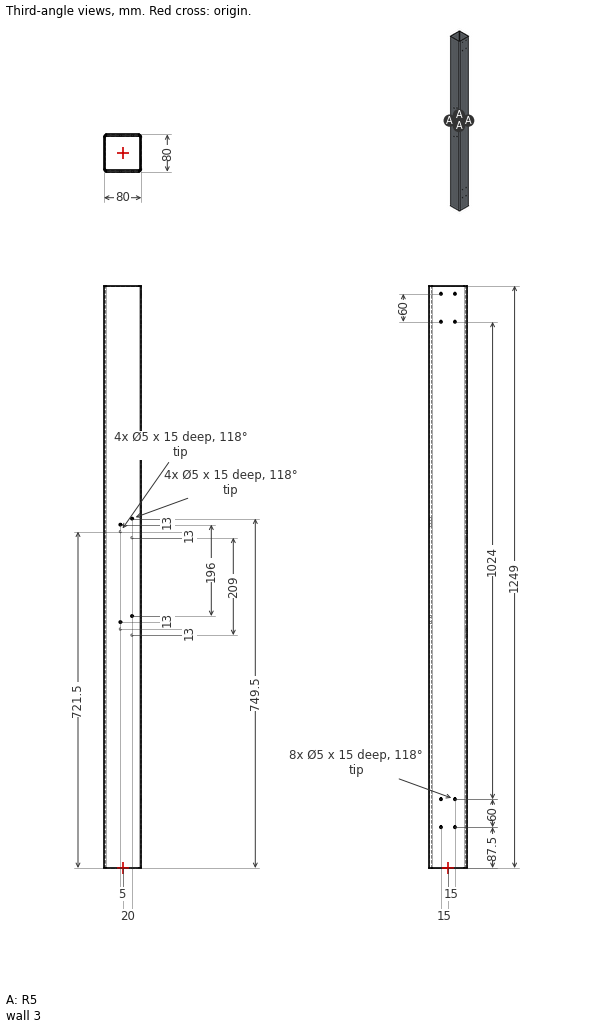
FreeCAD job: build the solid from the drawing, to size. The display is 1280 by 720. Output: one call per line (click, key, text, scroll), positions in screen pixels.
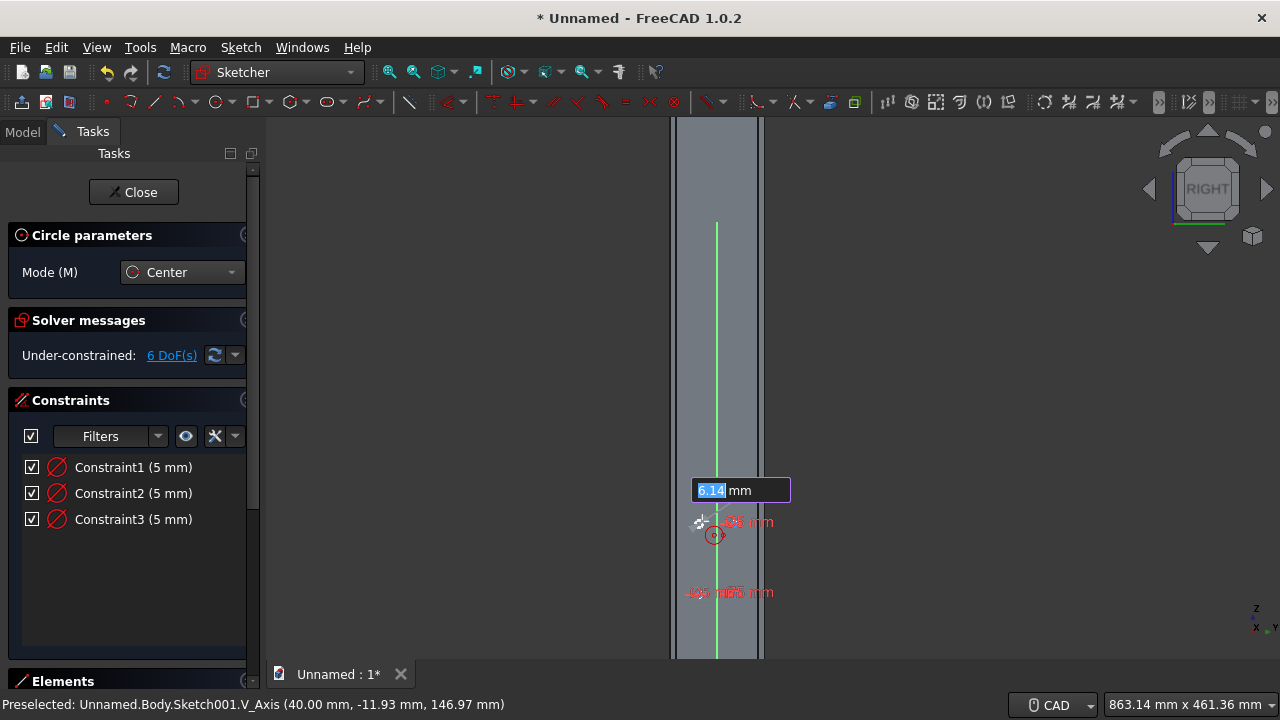
text(5)
key(Return)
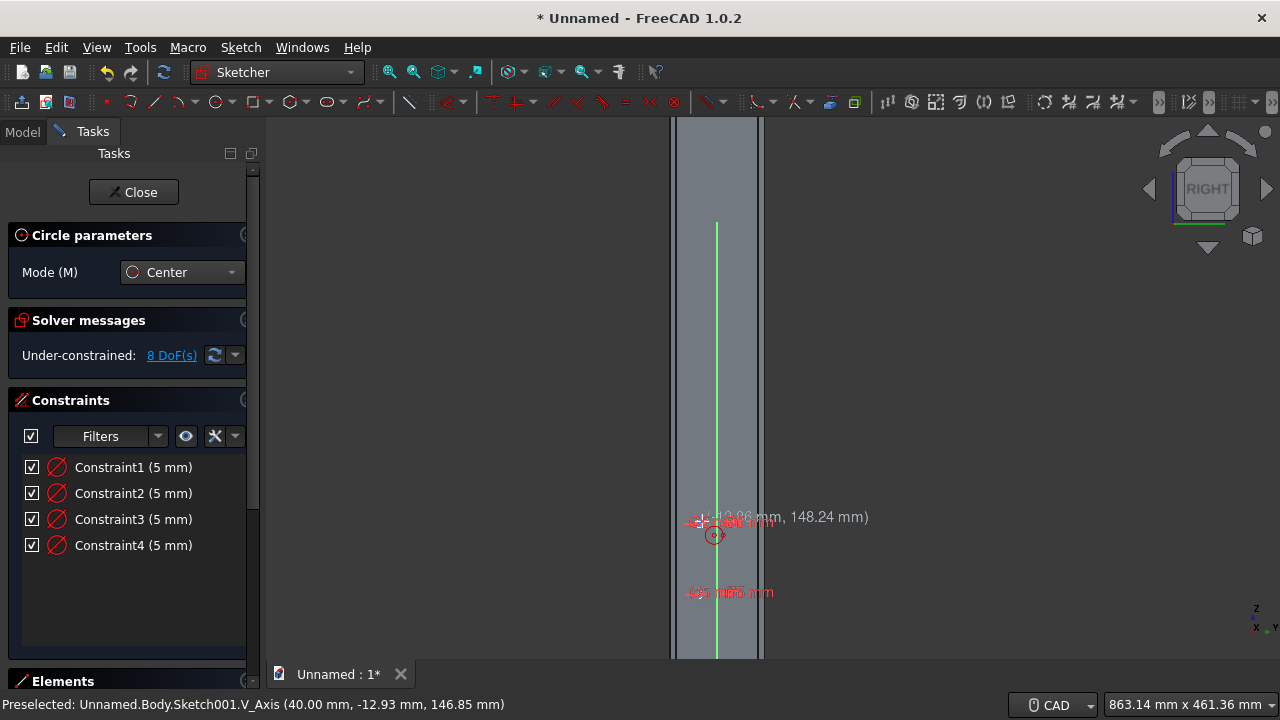
scroll(700, 524, down, 7)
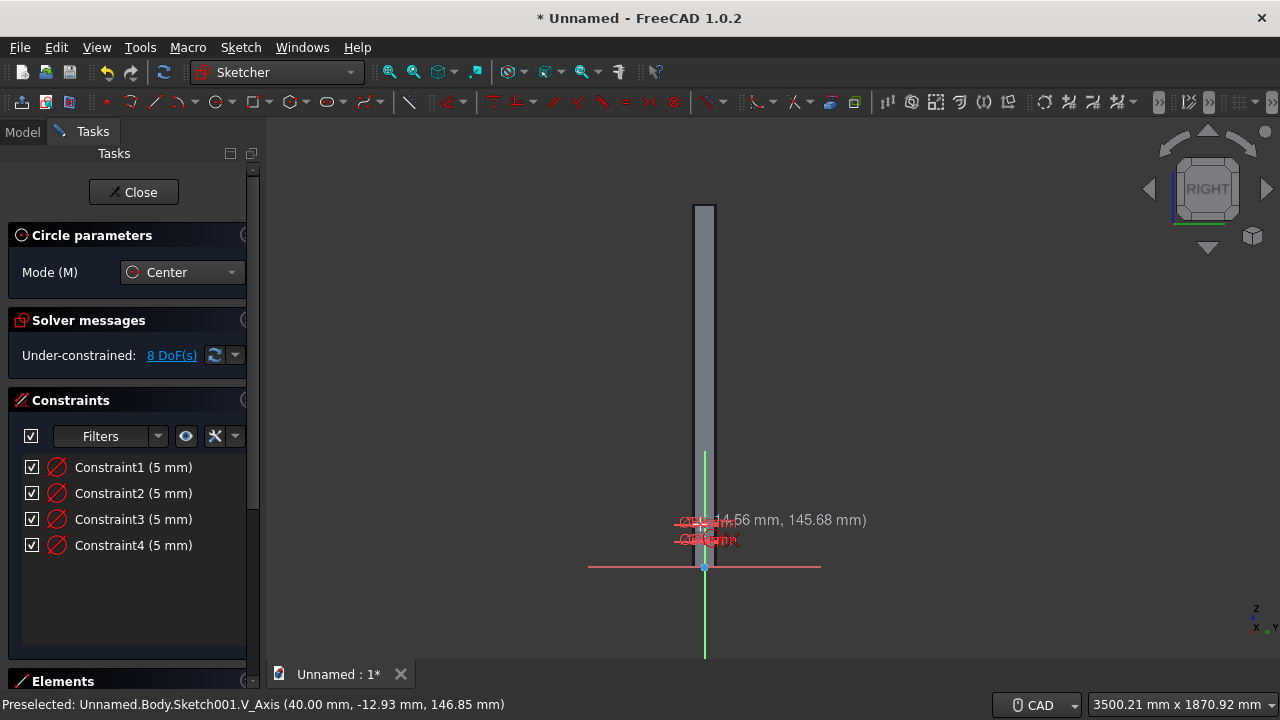
scroll(709, 228, up, 18)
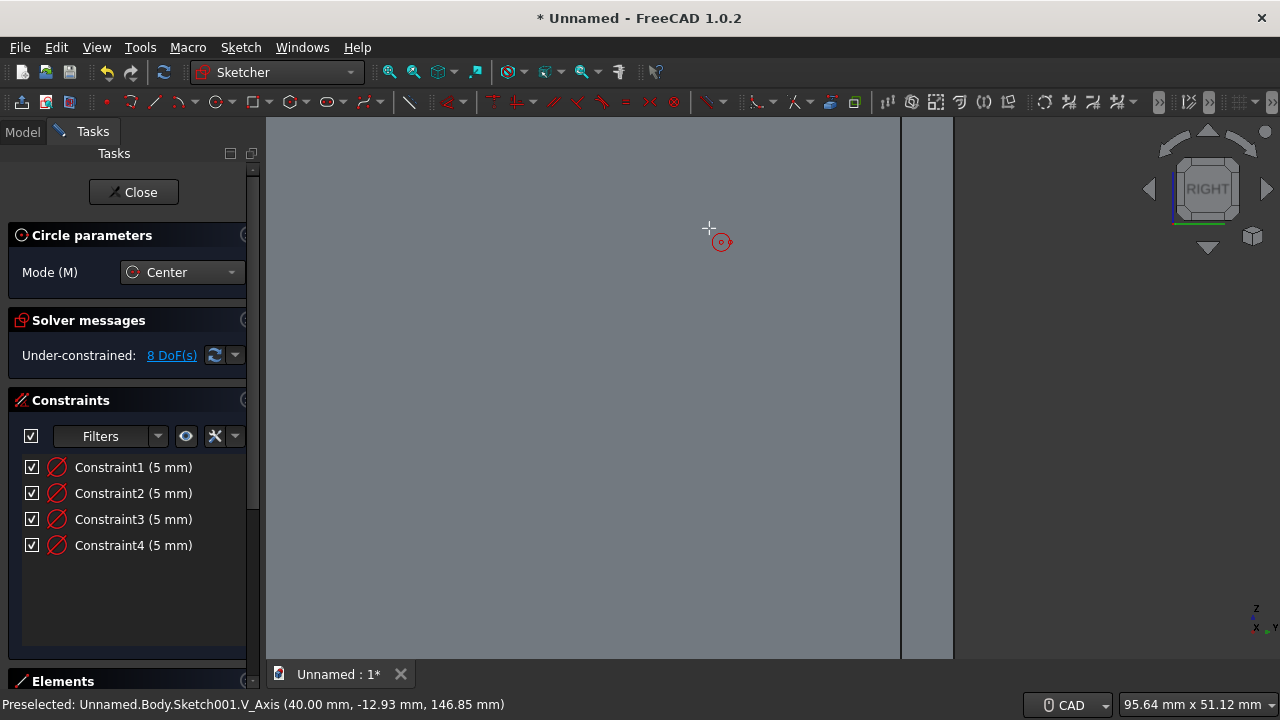
scroll(709, 228, down, 18)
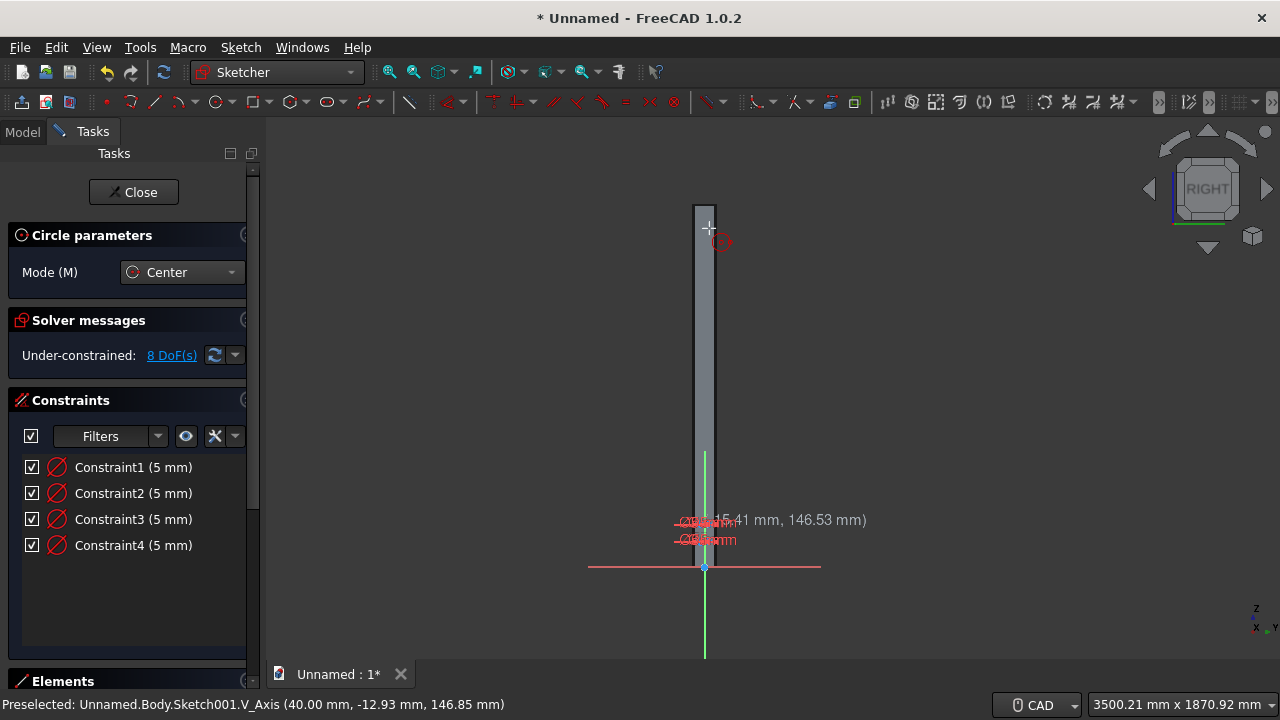
scroll(709, 228, up, 7)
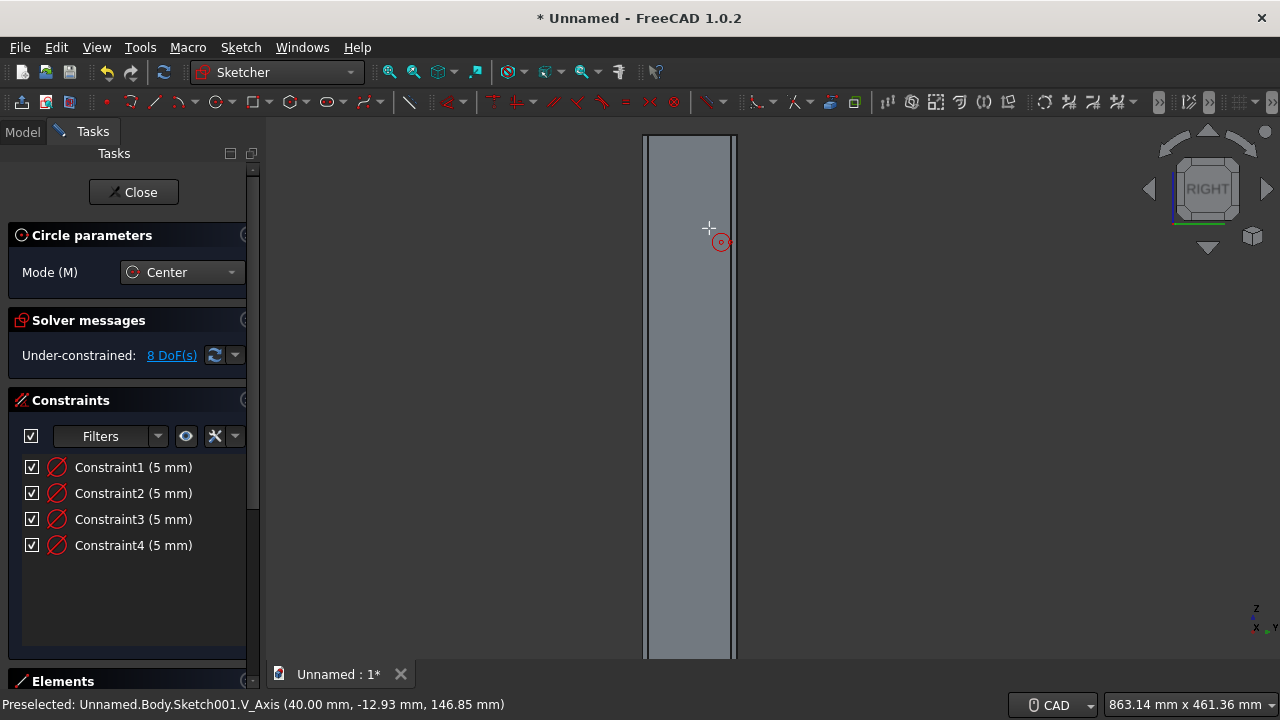
click(707, 226)
move(709, 224)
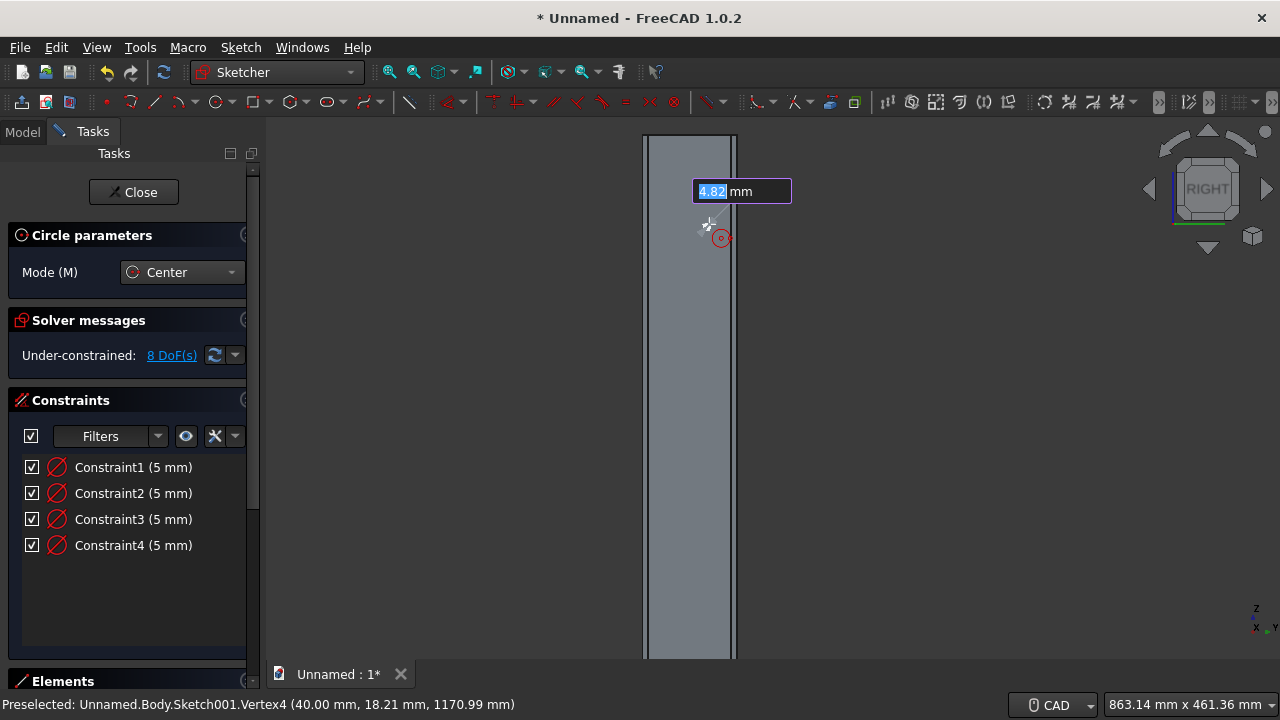
text(5)
key(Return)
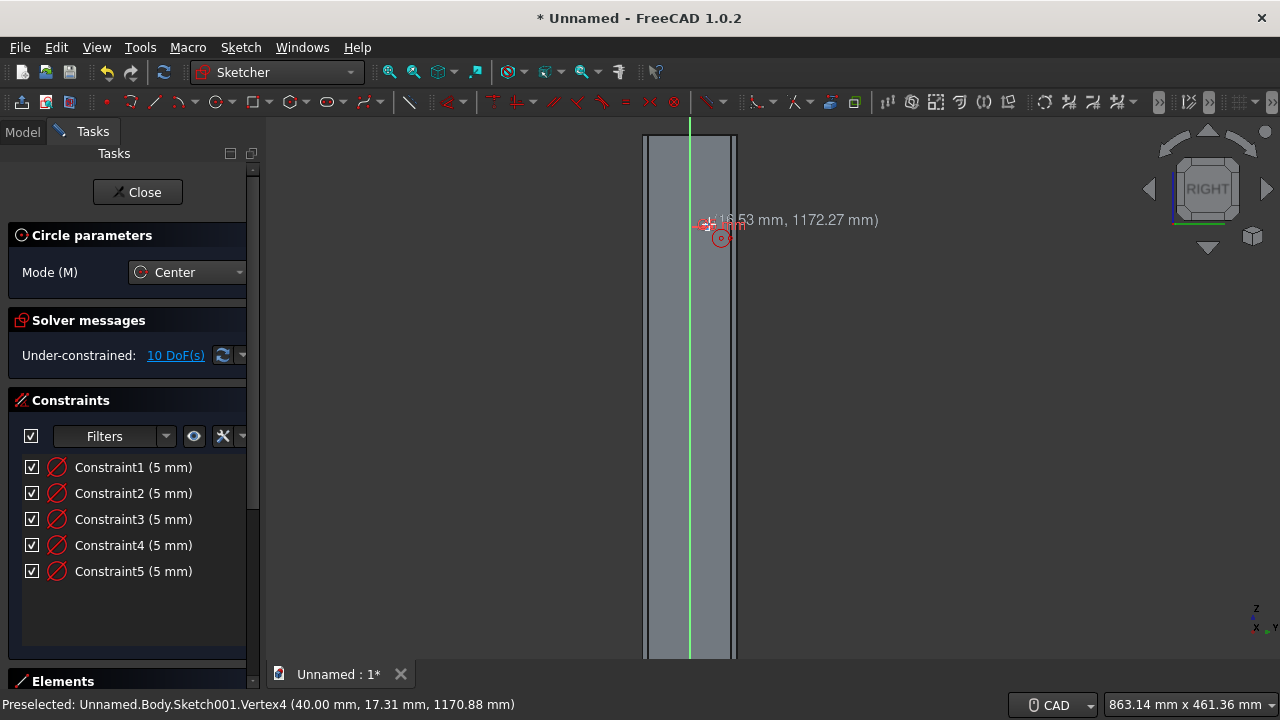
scroll(672, 226, up, 11)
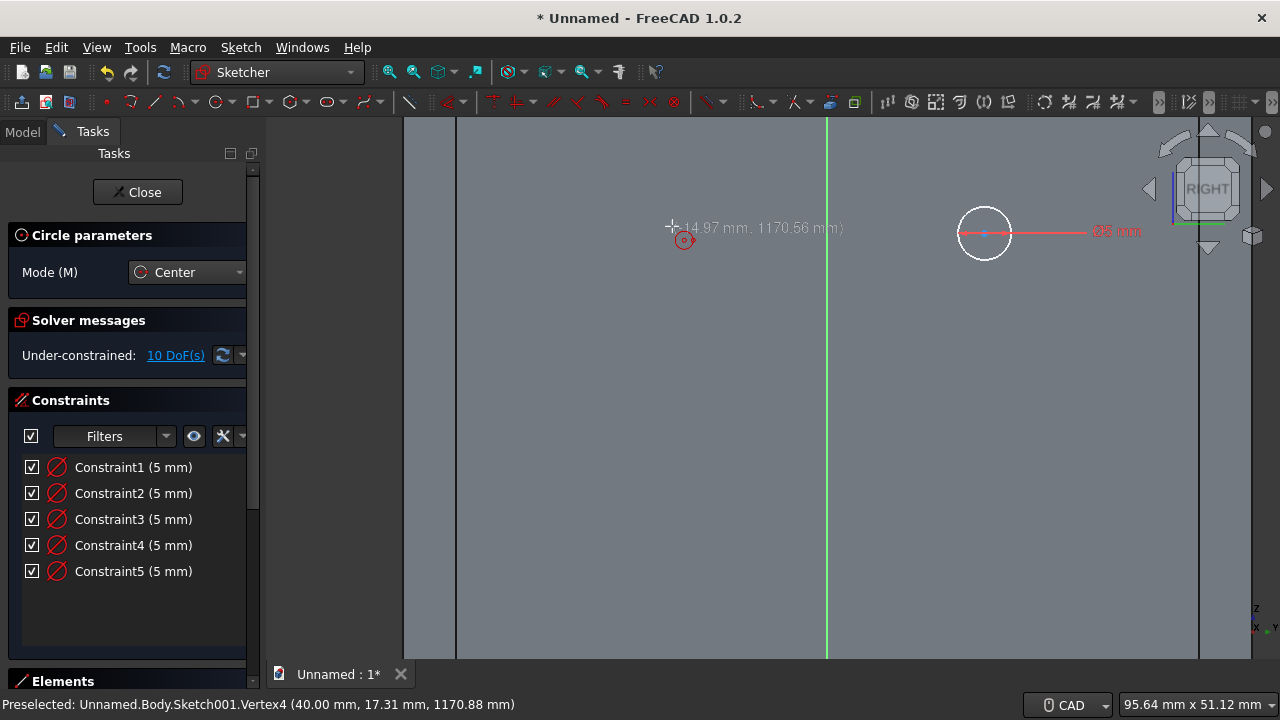
scroll(701, 227, down, 18)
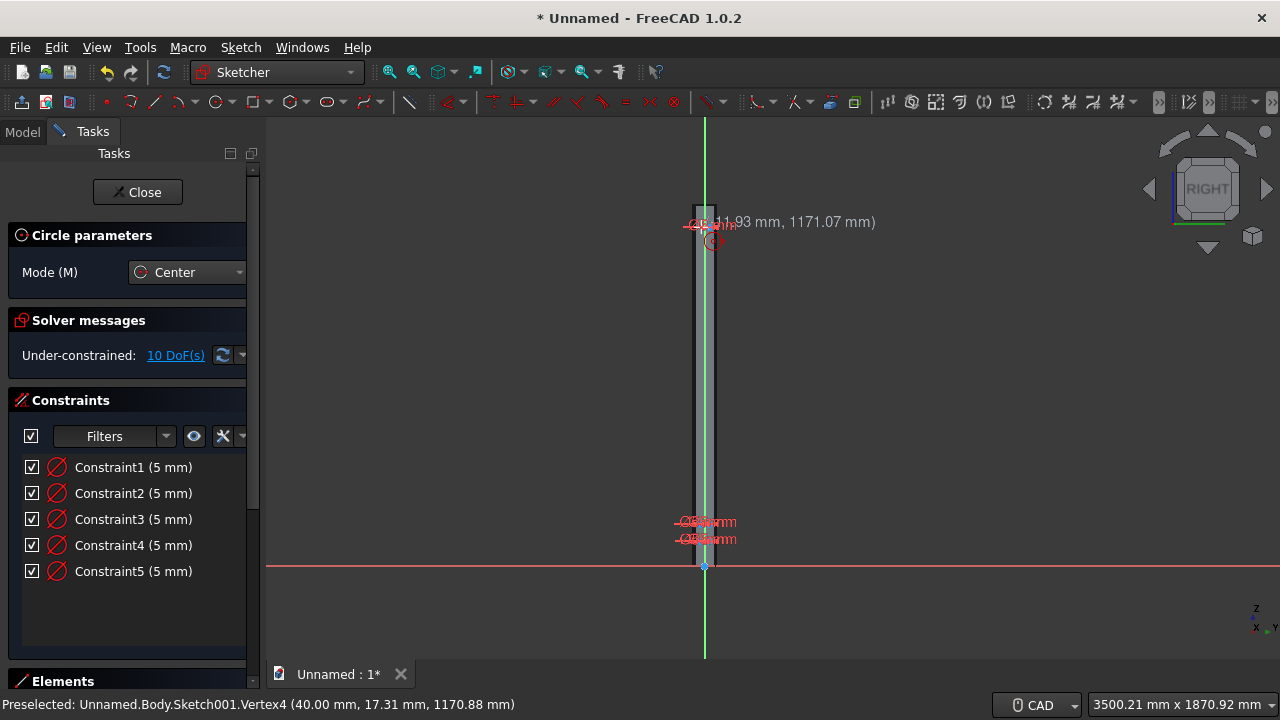
scroll(701, 227, up, 7)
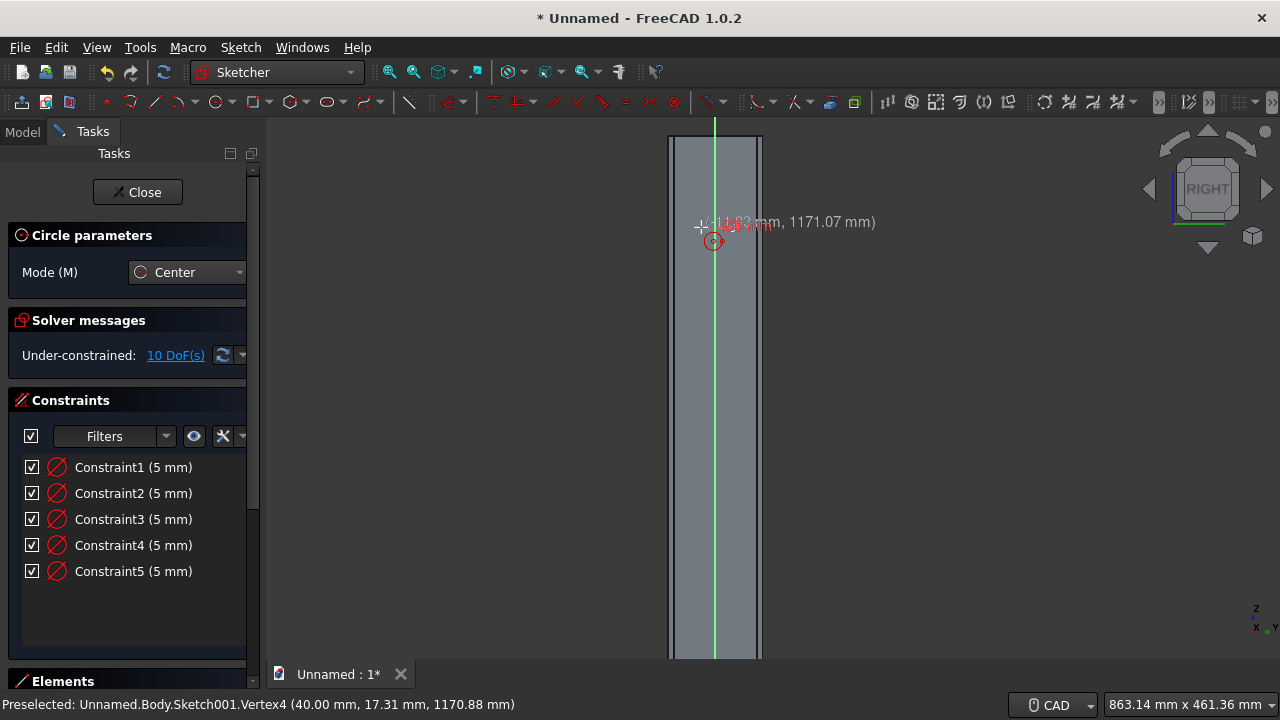
click(698, 227)
move(700, 225)